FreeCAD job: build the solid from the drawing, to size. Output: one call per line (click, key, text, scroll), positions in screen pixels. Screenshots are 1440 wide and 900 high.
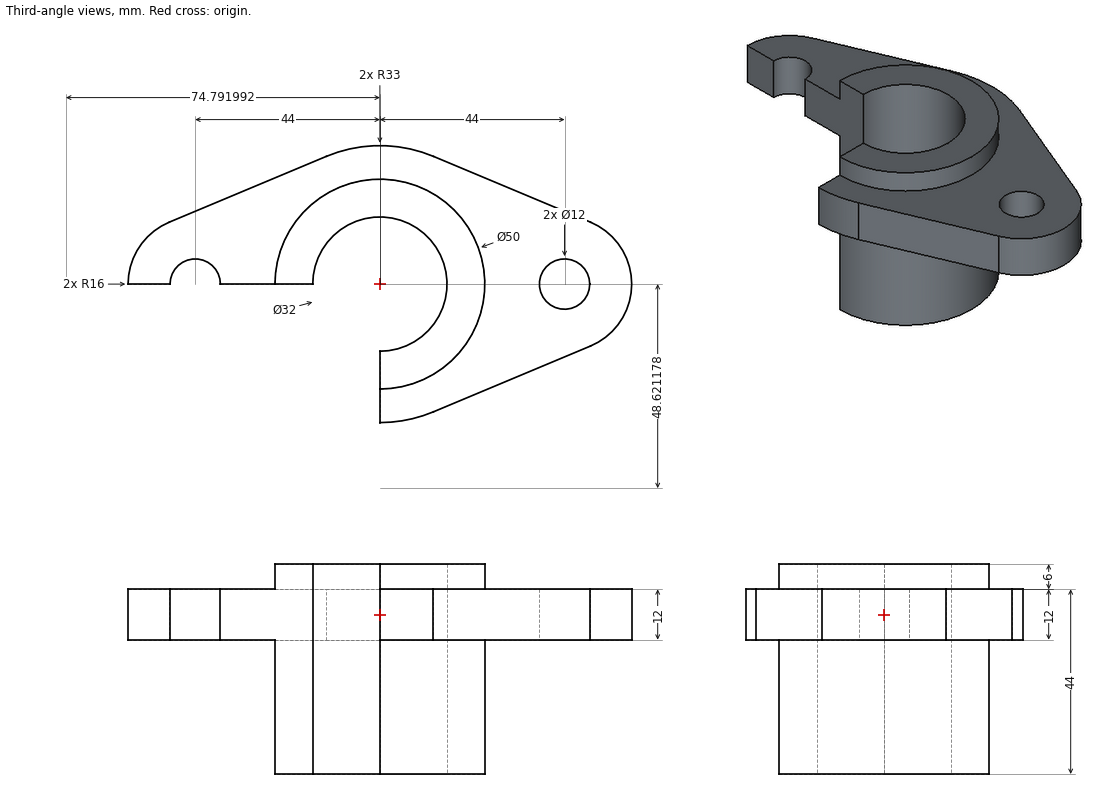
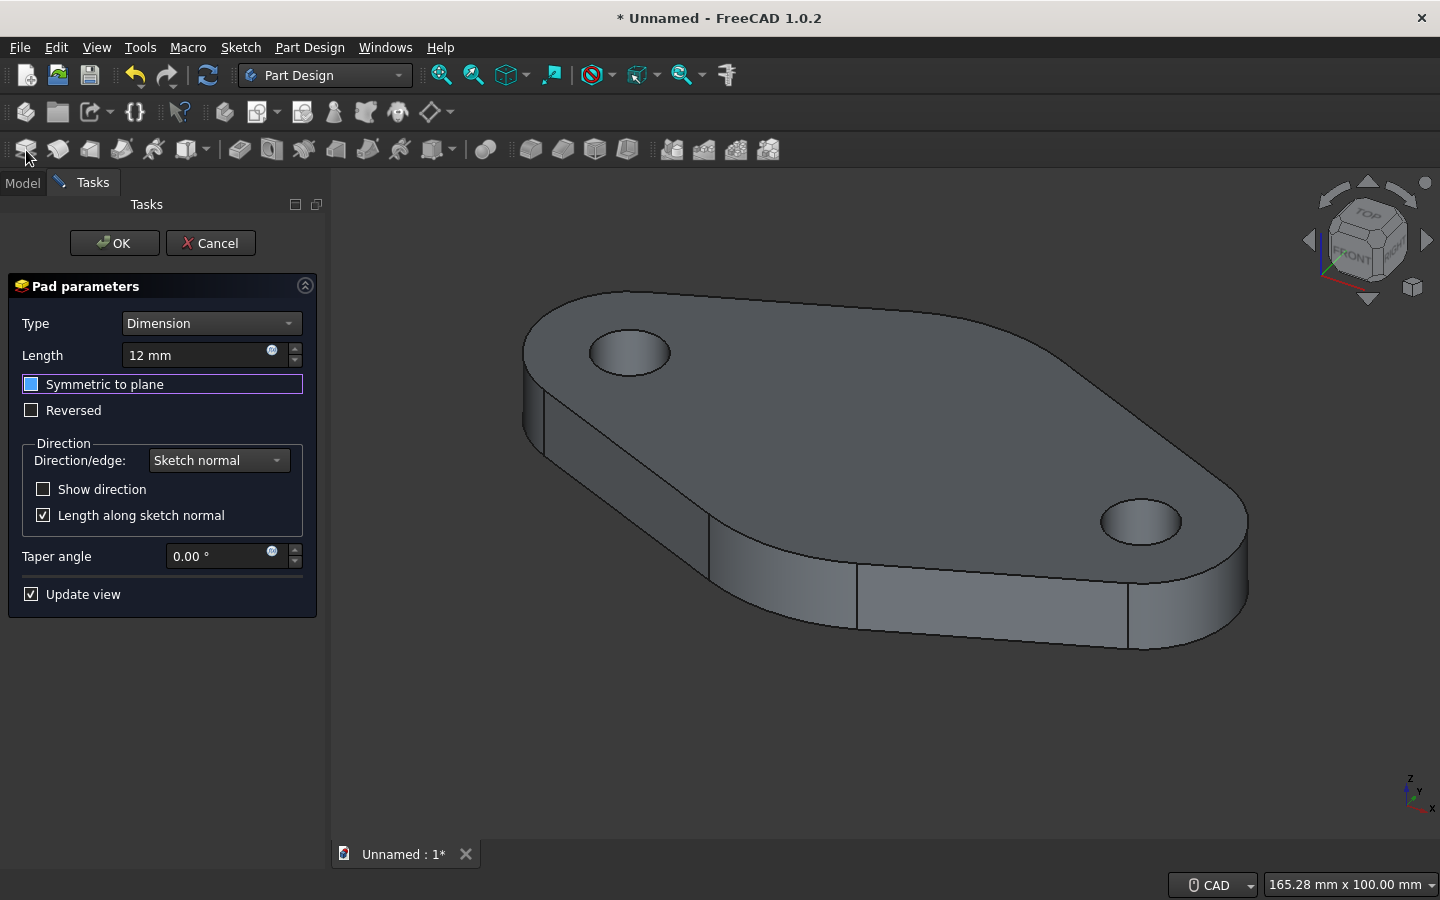
click(30, 384)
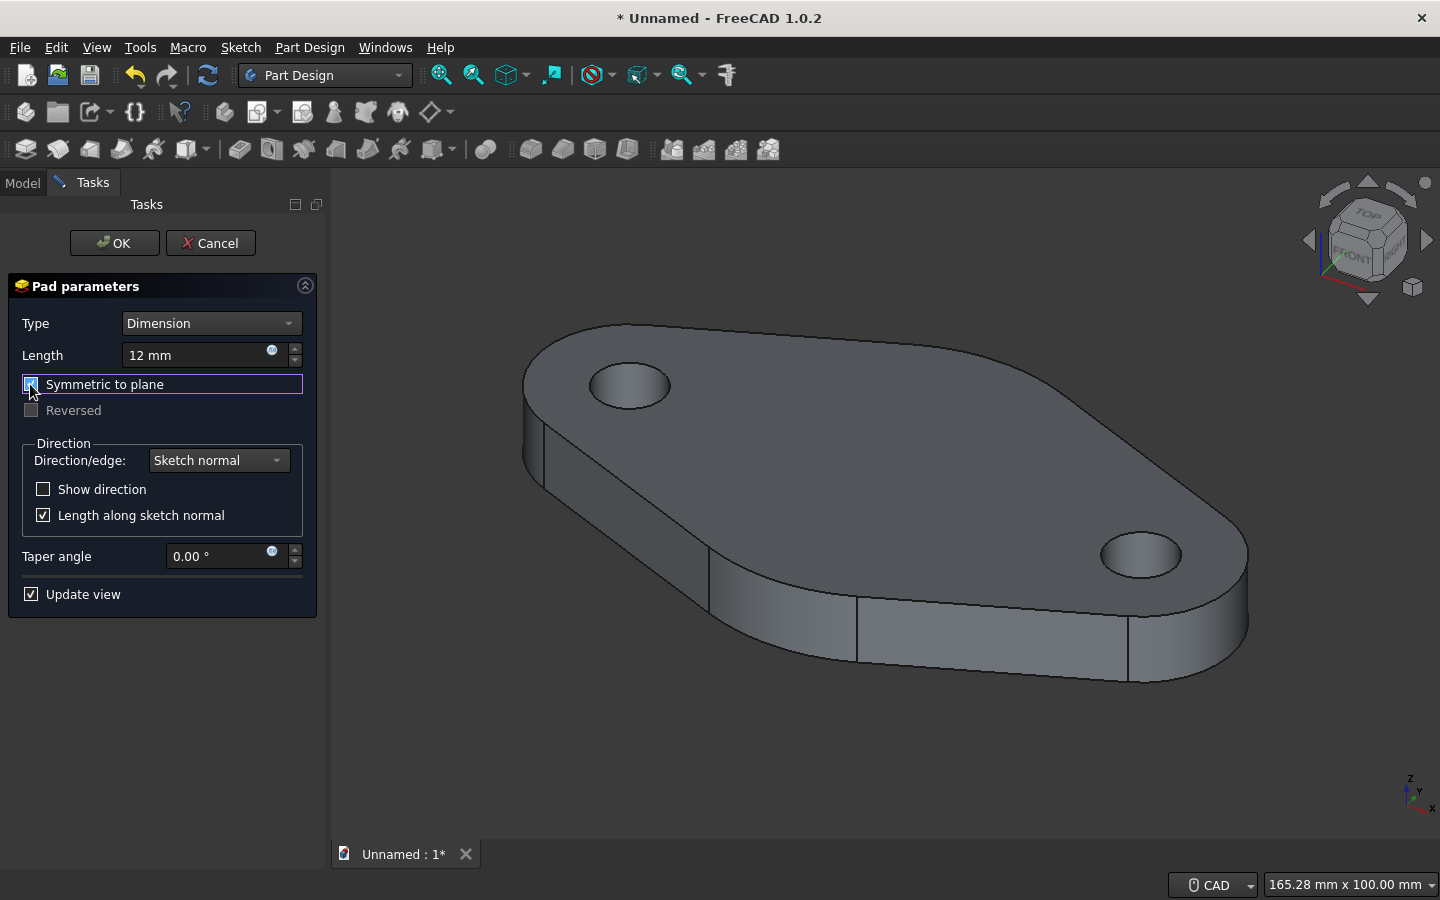
click(115, 243)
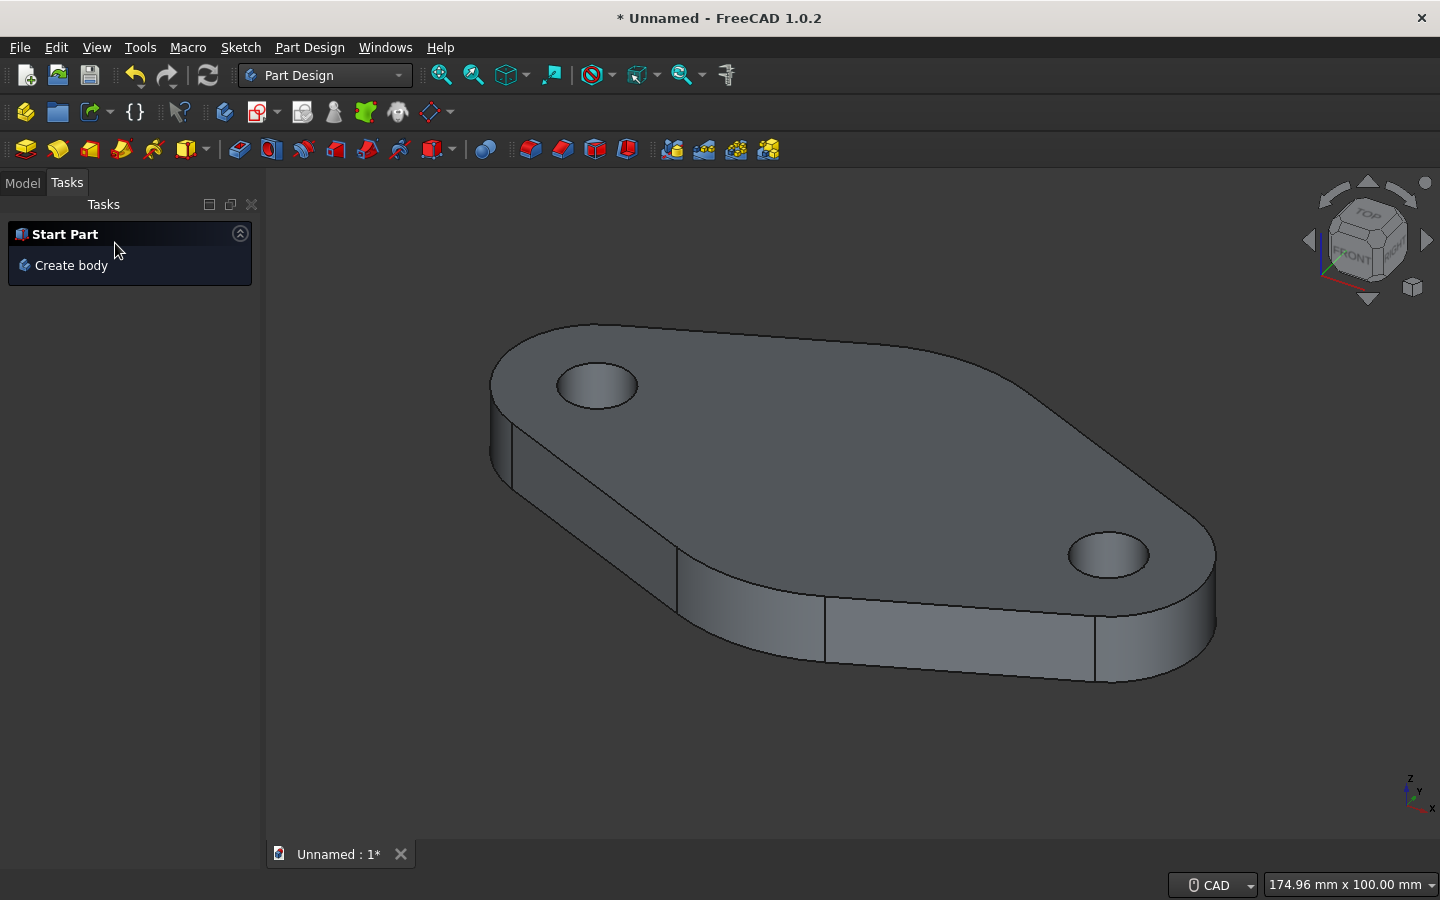
click(853, 470)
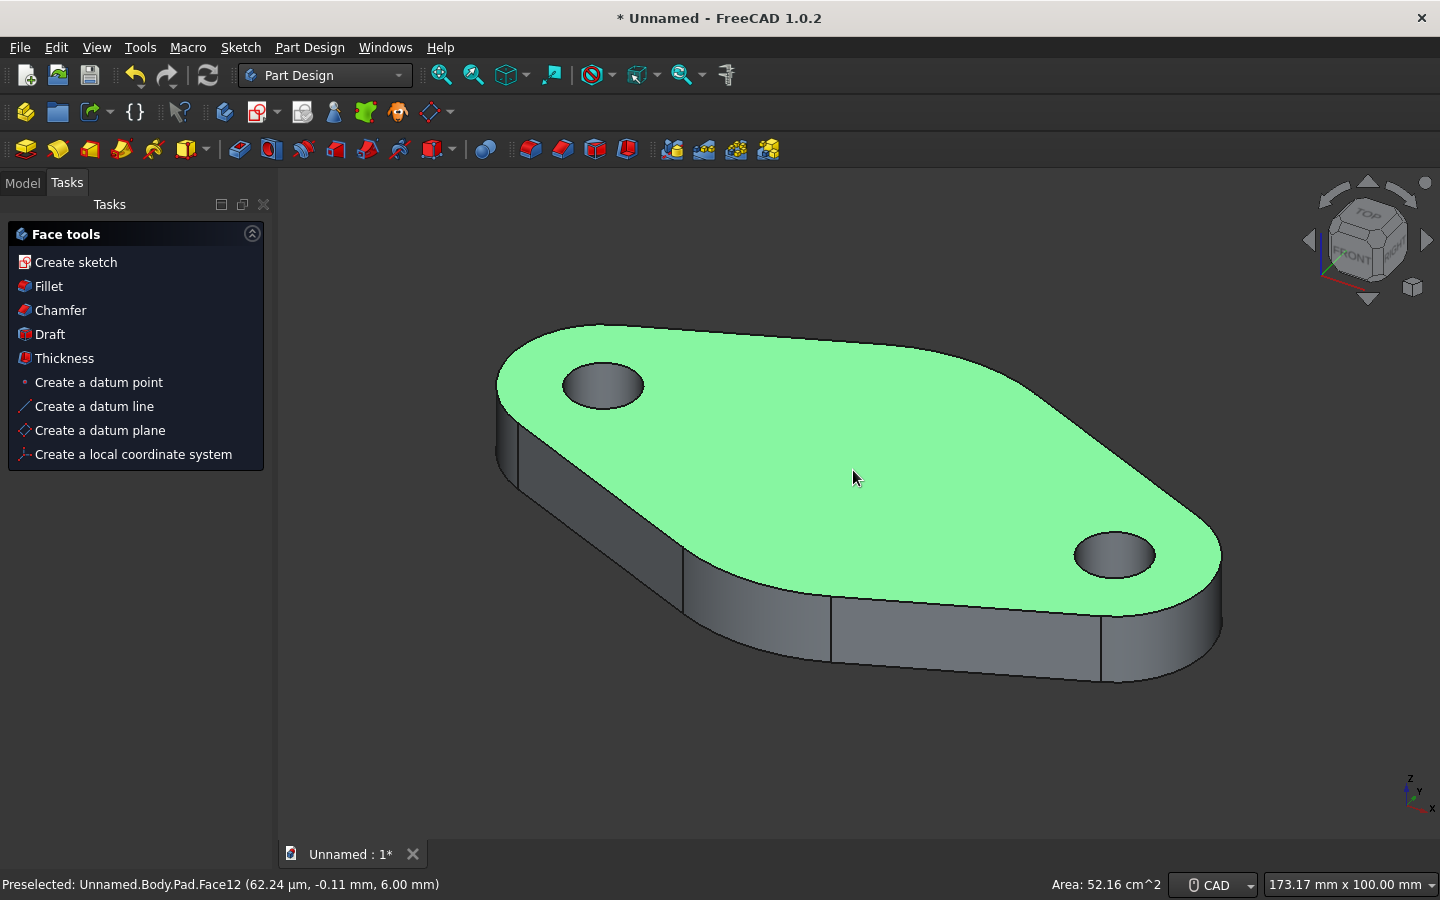
click(258, 112)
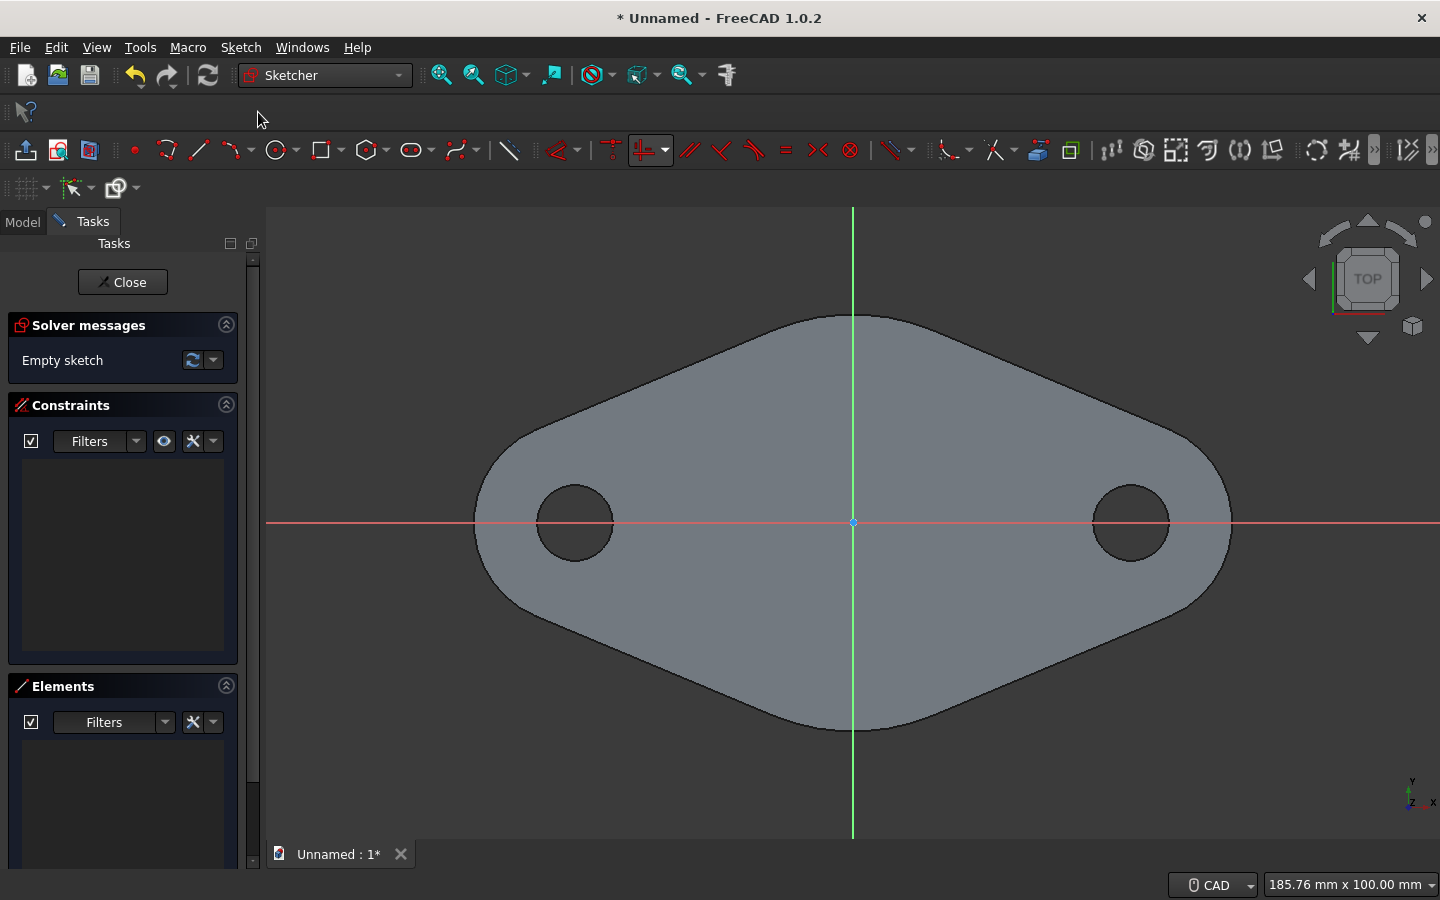
scroll(936, 523, up, 3)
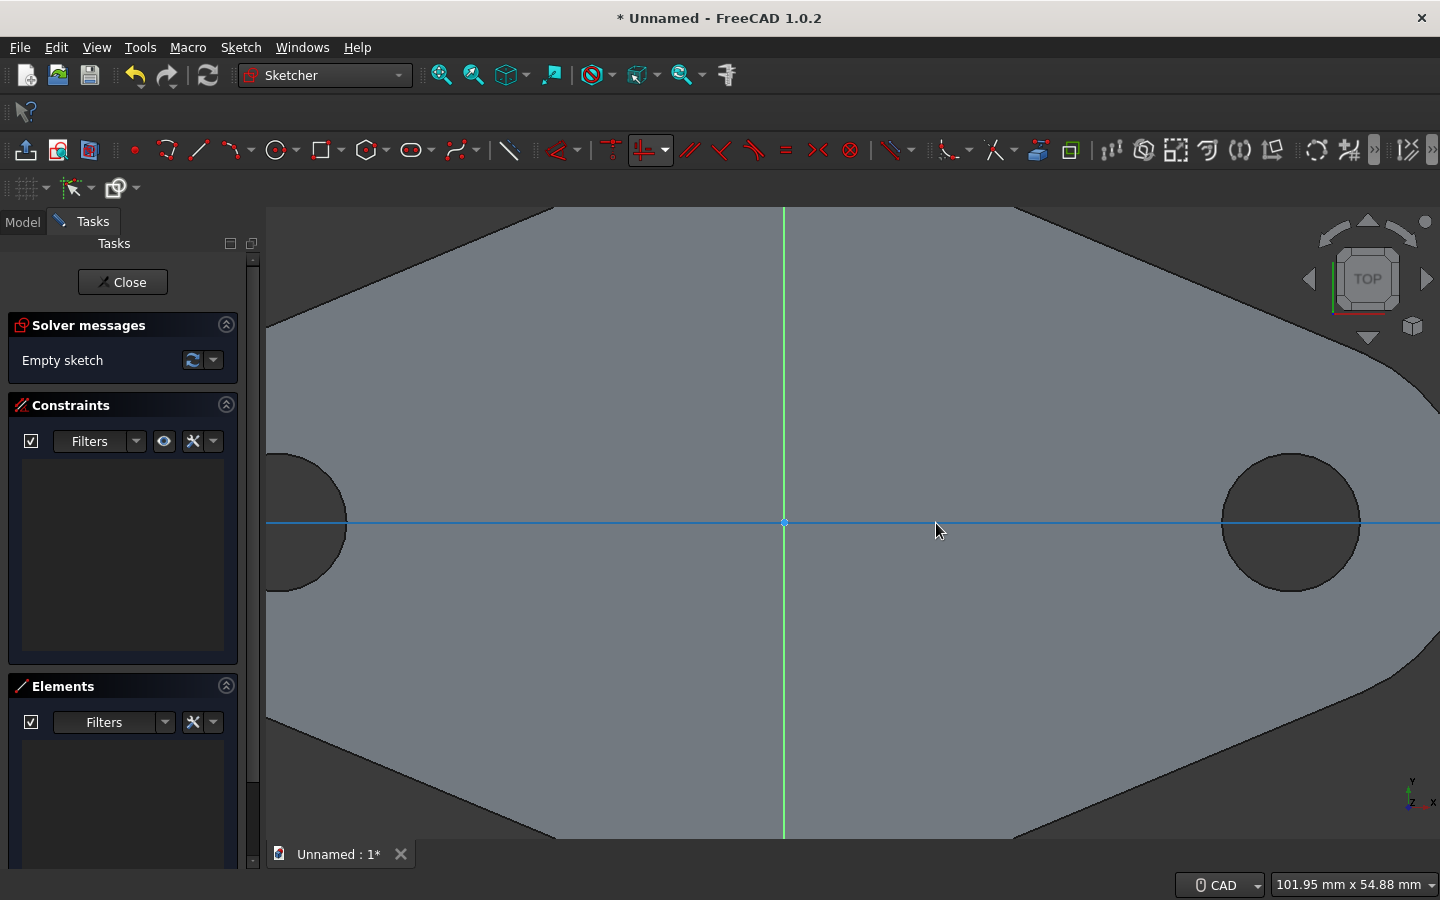
click(276, 150)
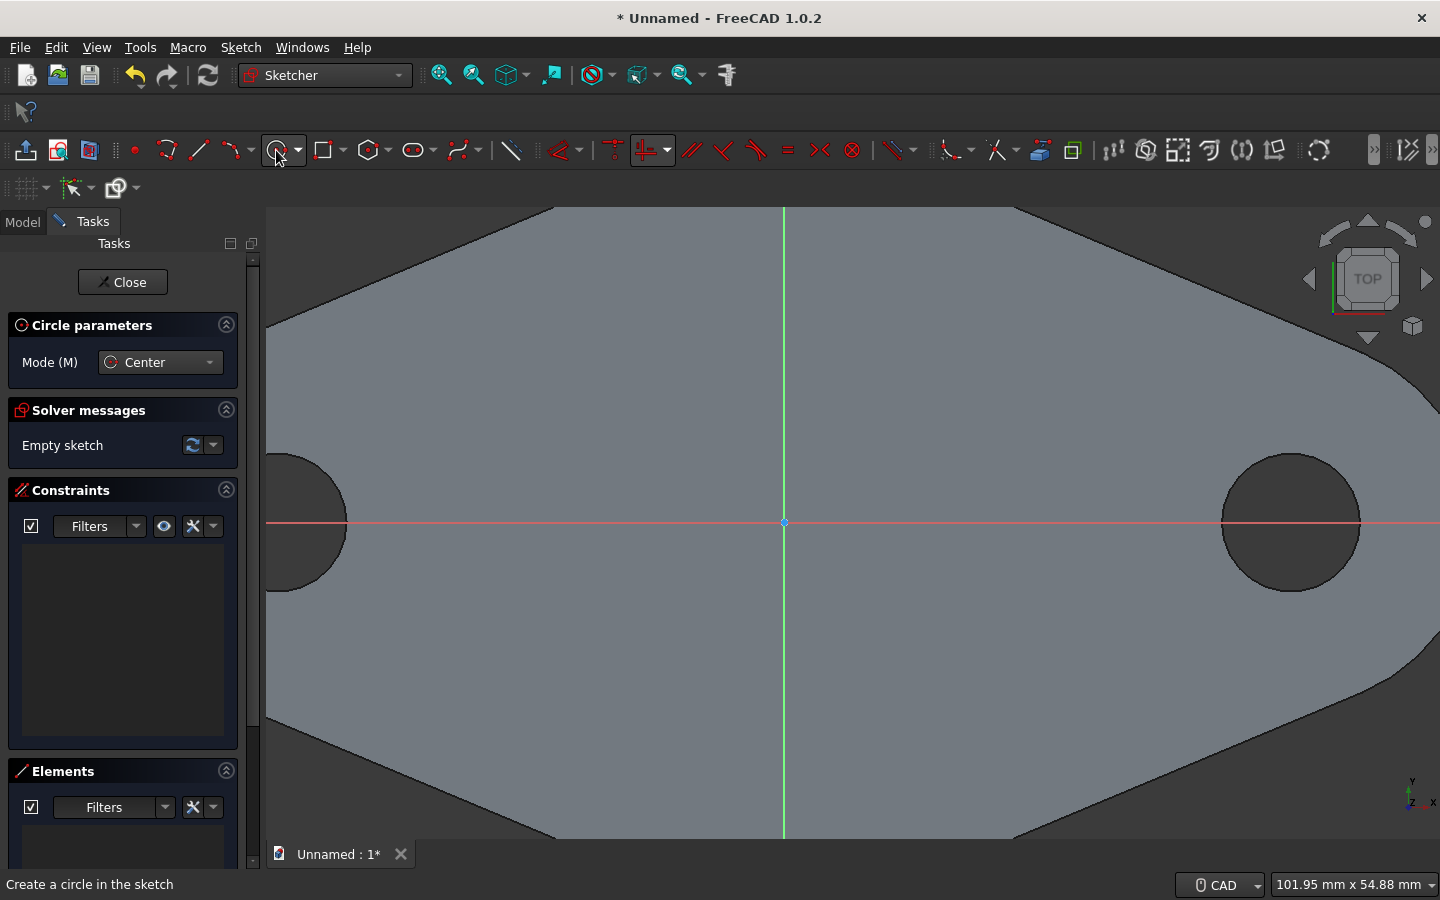
click(784, 523)
move(915, 392)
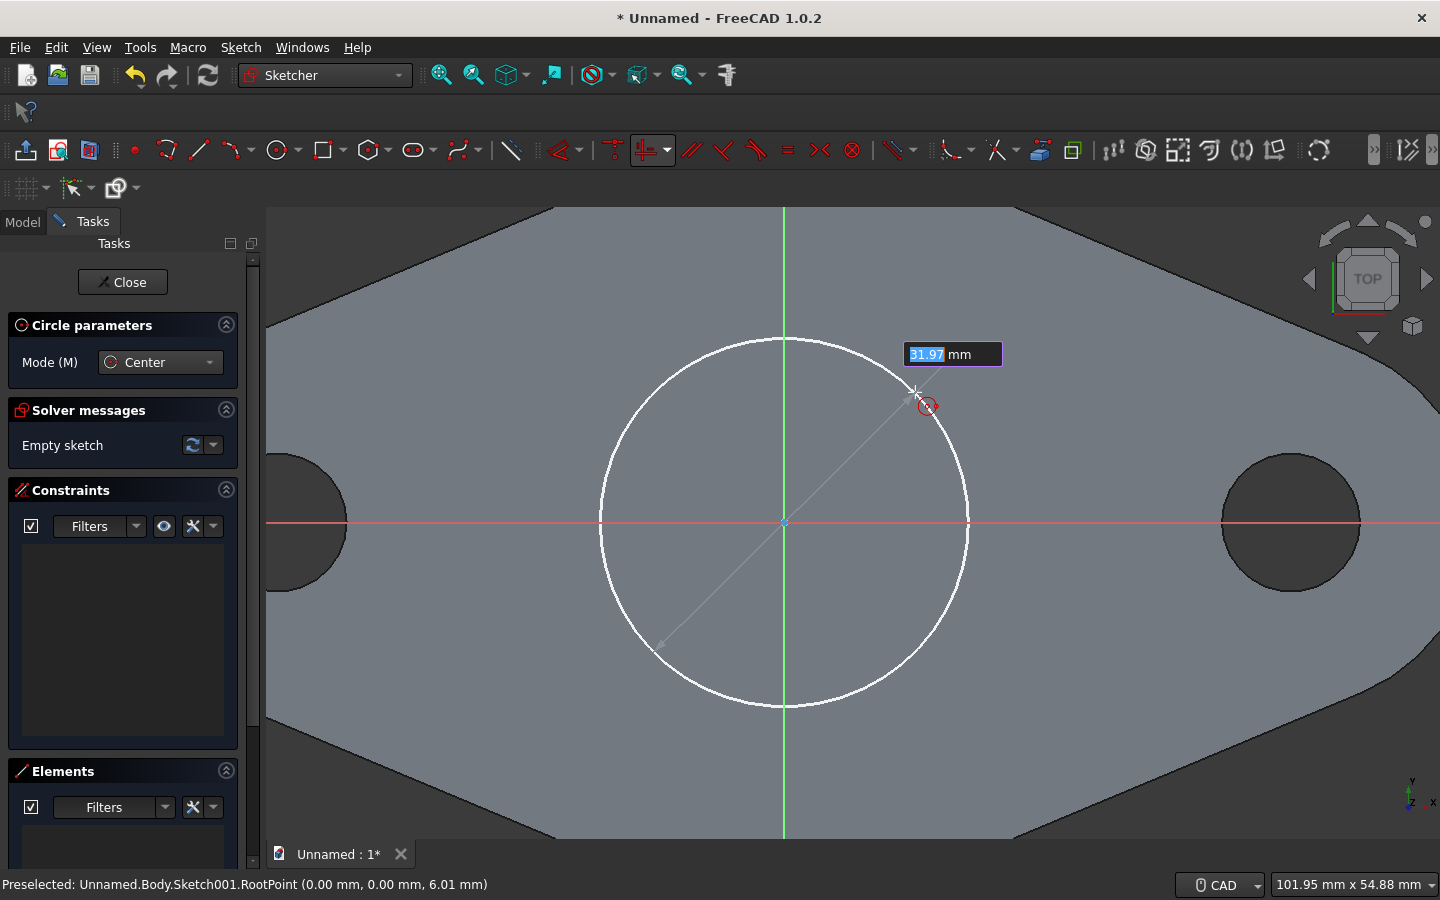
text(32)
key(Return)
key(Escape)